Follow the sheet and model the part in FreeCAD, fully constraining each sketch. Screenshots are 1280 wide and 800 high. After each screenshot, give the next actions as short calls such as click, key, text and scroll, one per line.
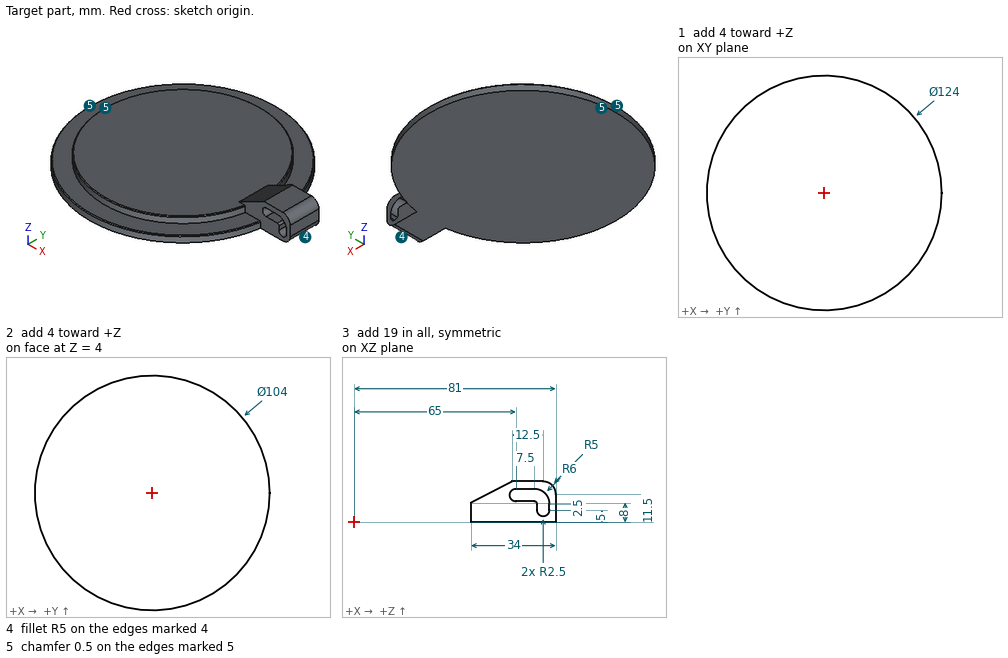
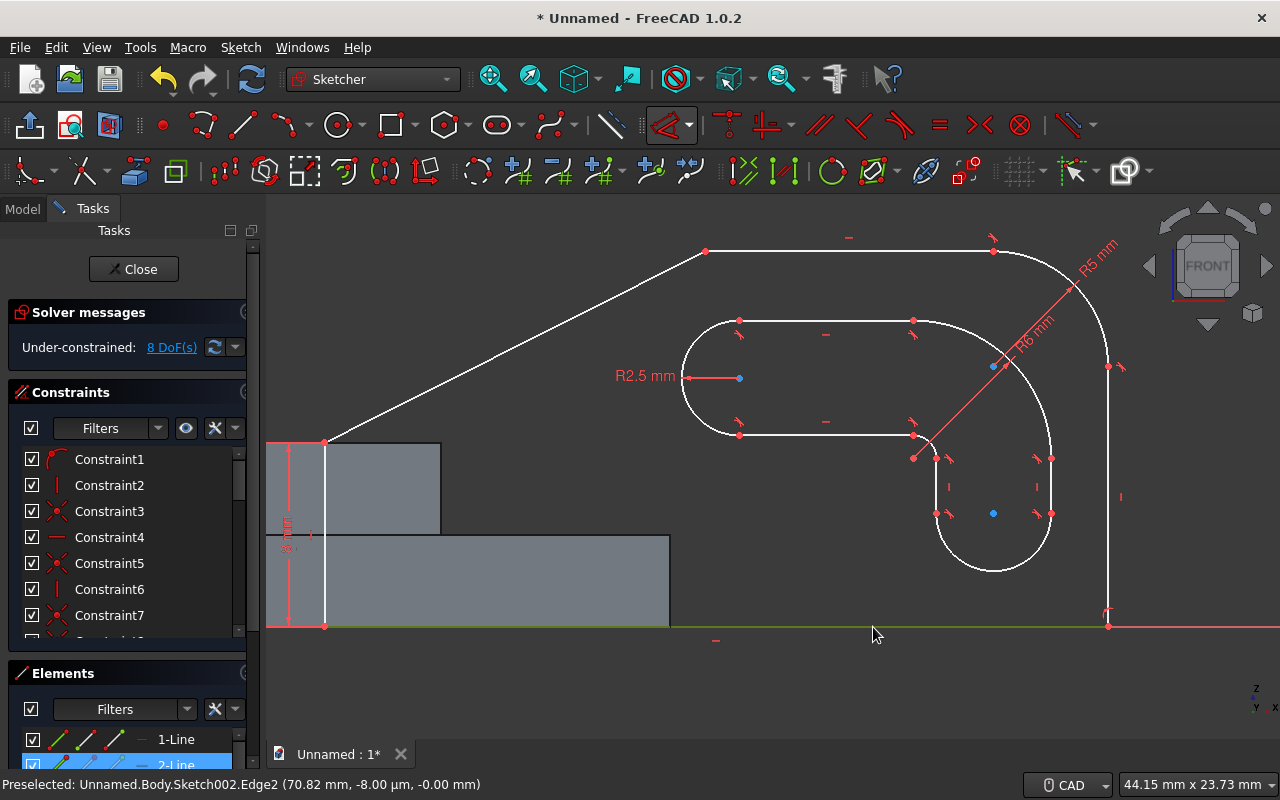
key(l)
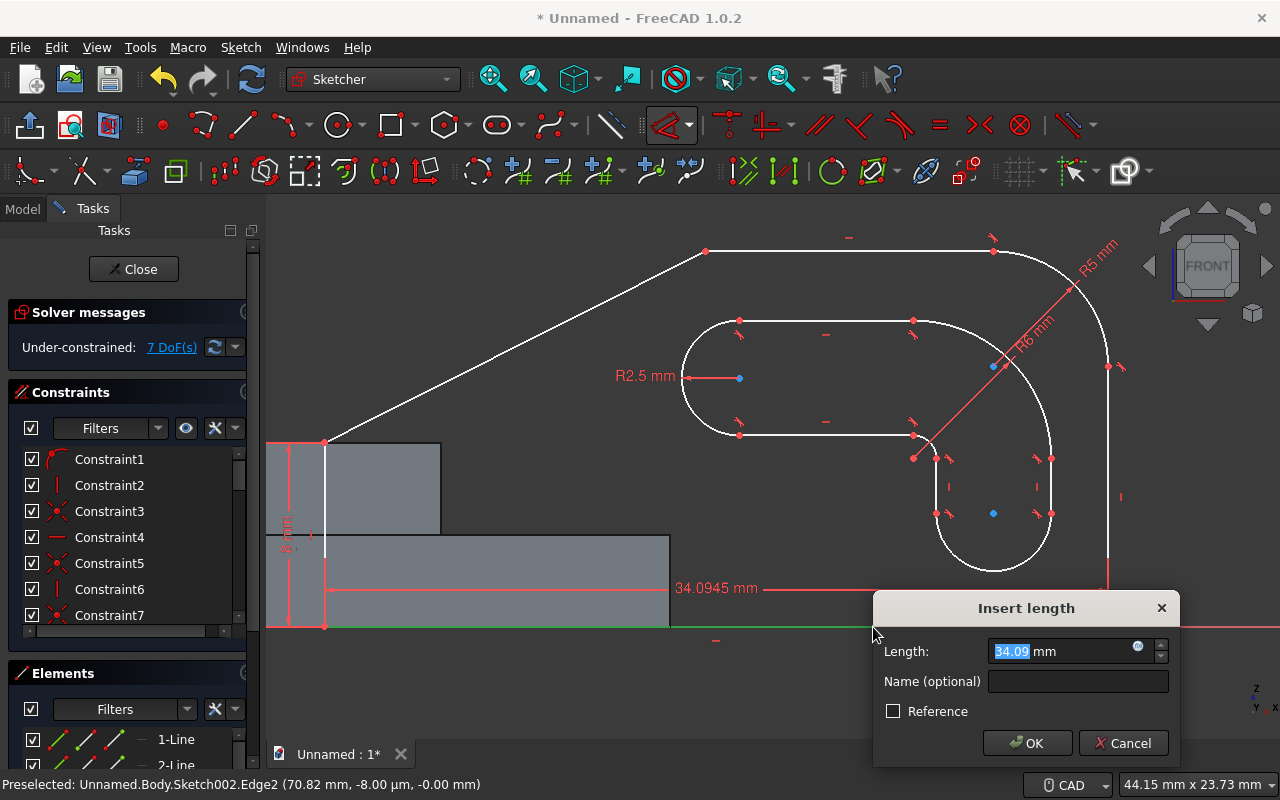
text(34)
key(Return)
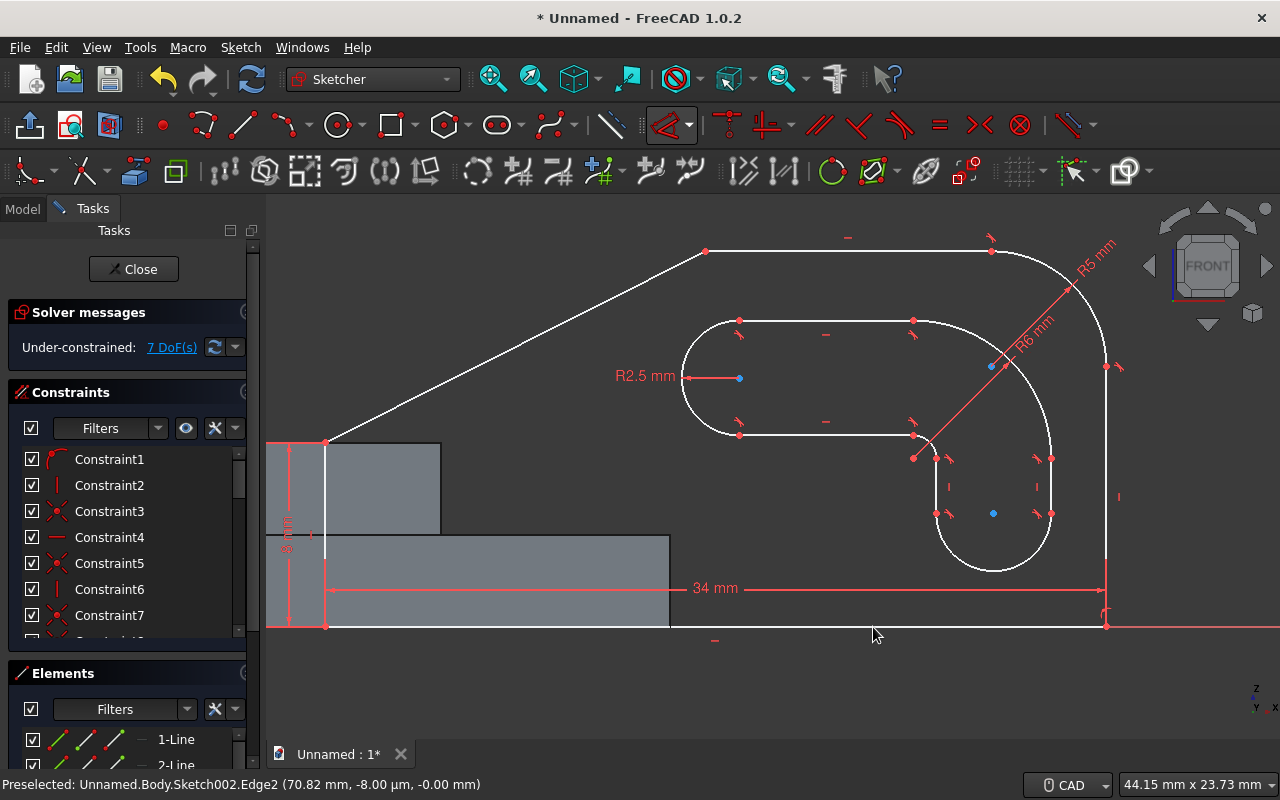
click(1051, 514)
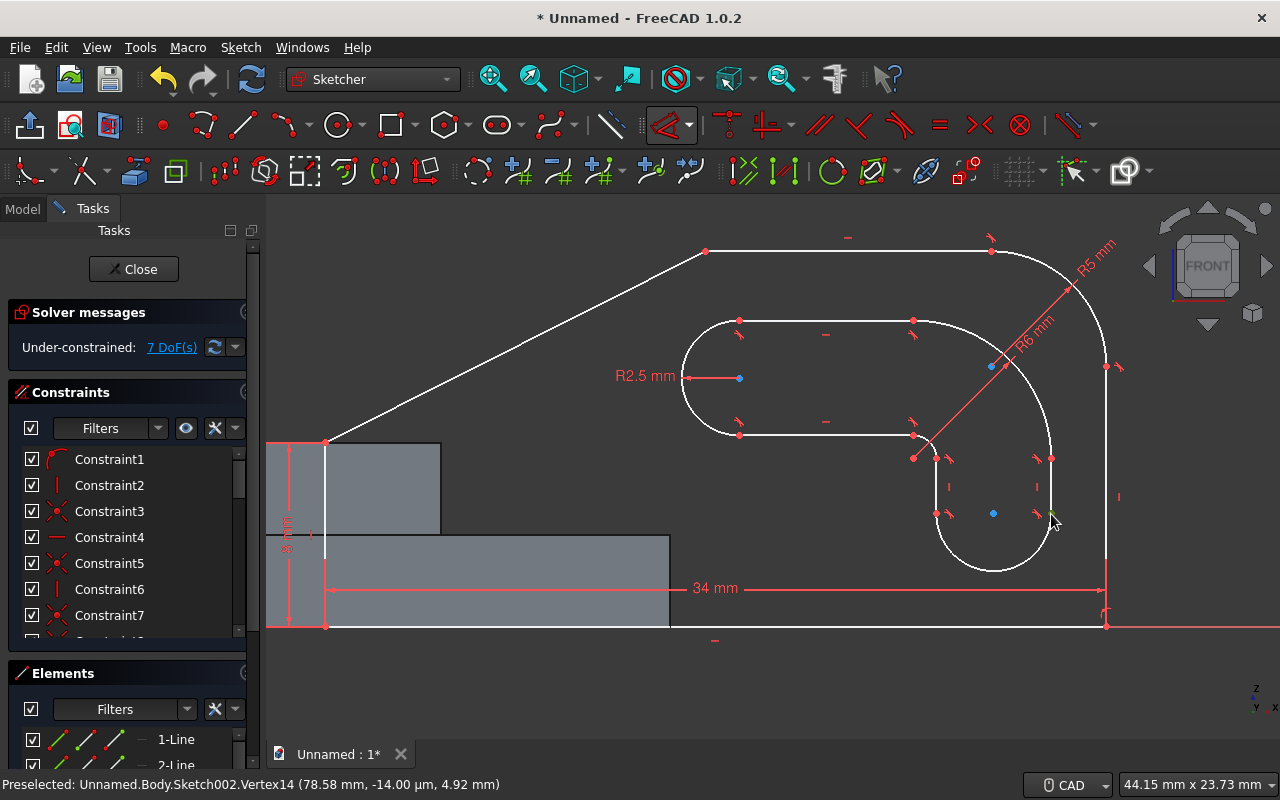
click(692, 126)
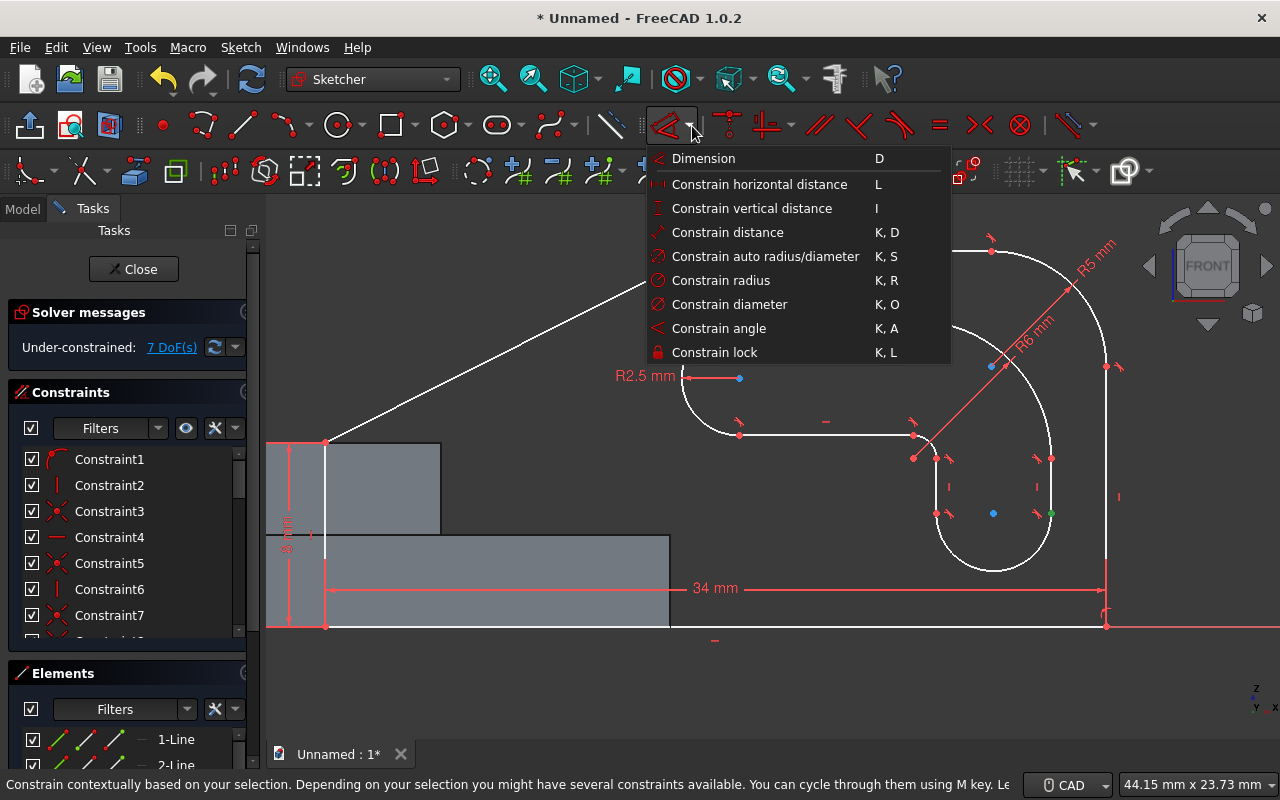
click(799, 208)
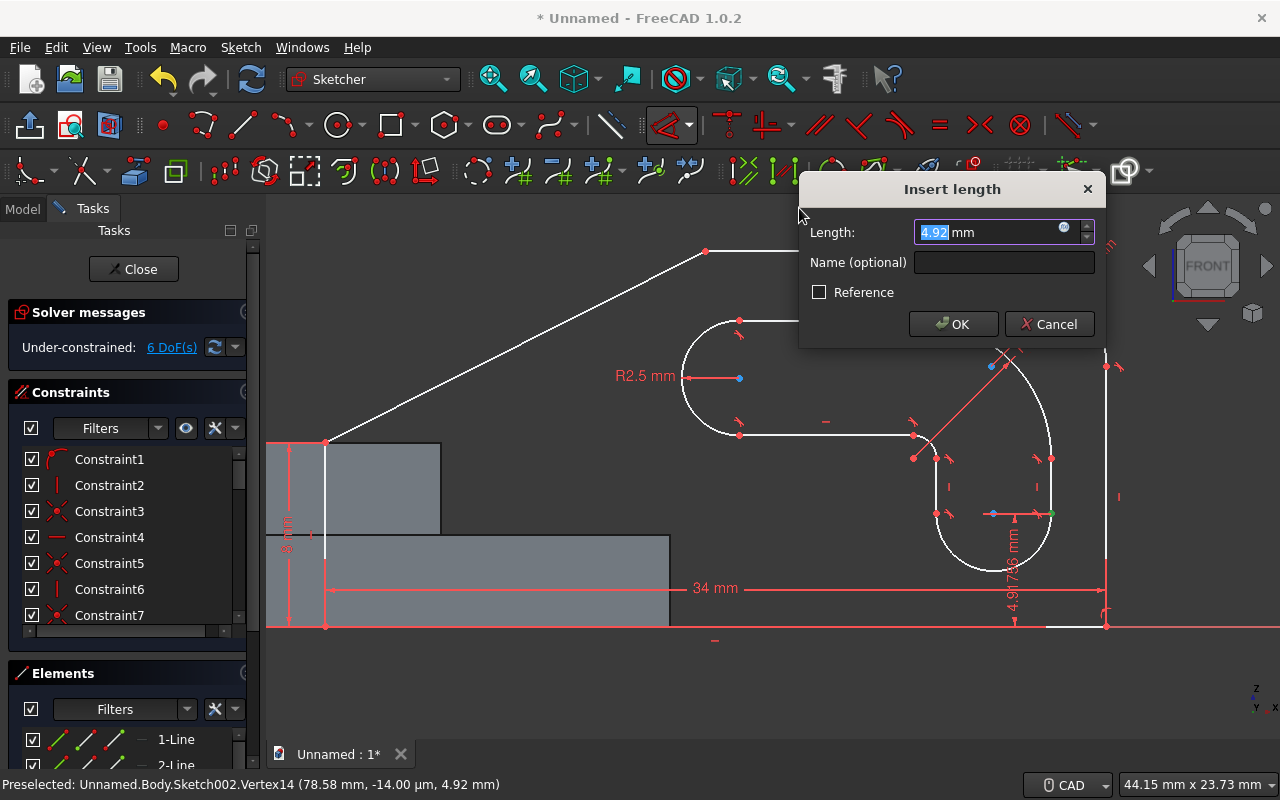
text(5)
key(Return)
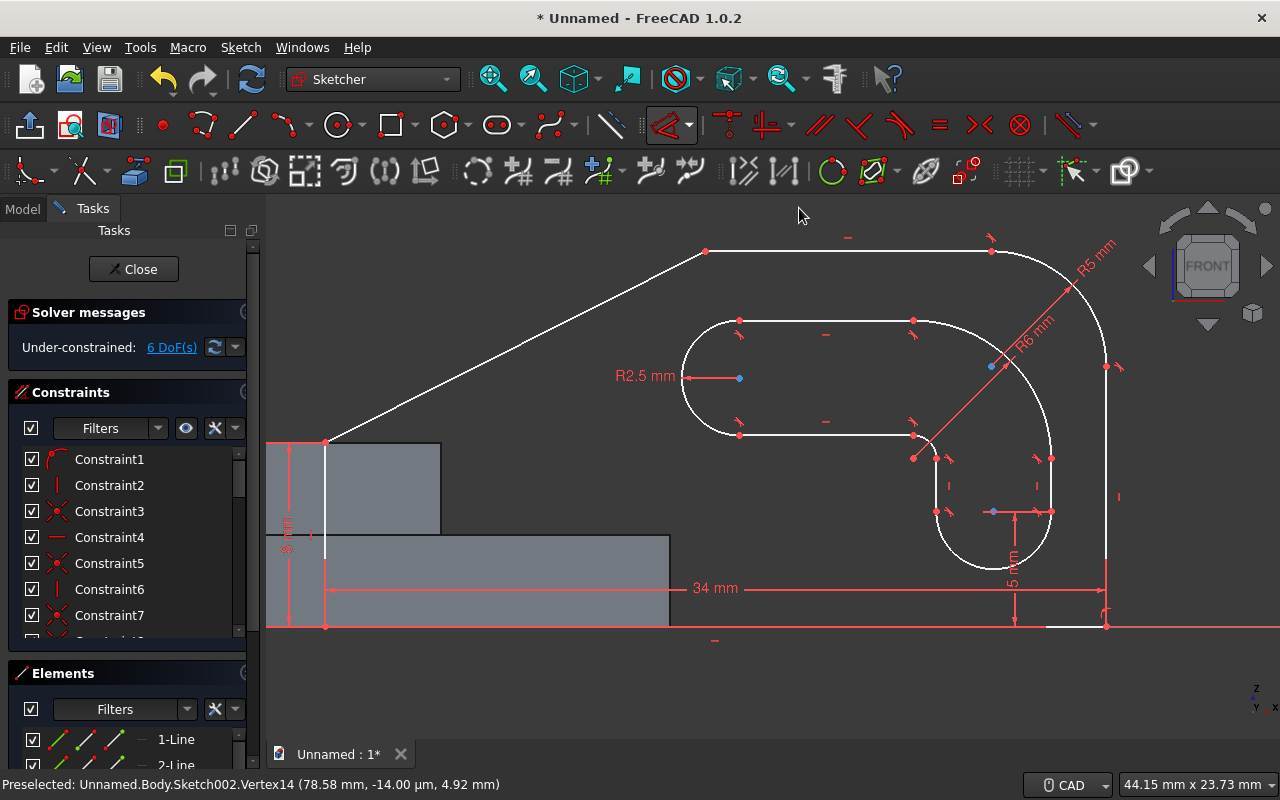
click(1051, 496)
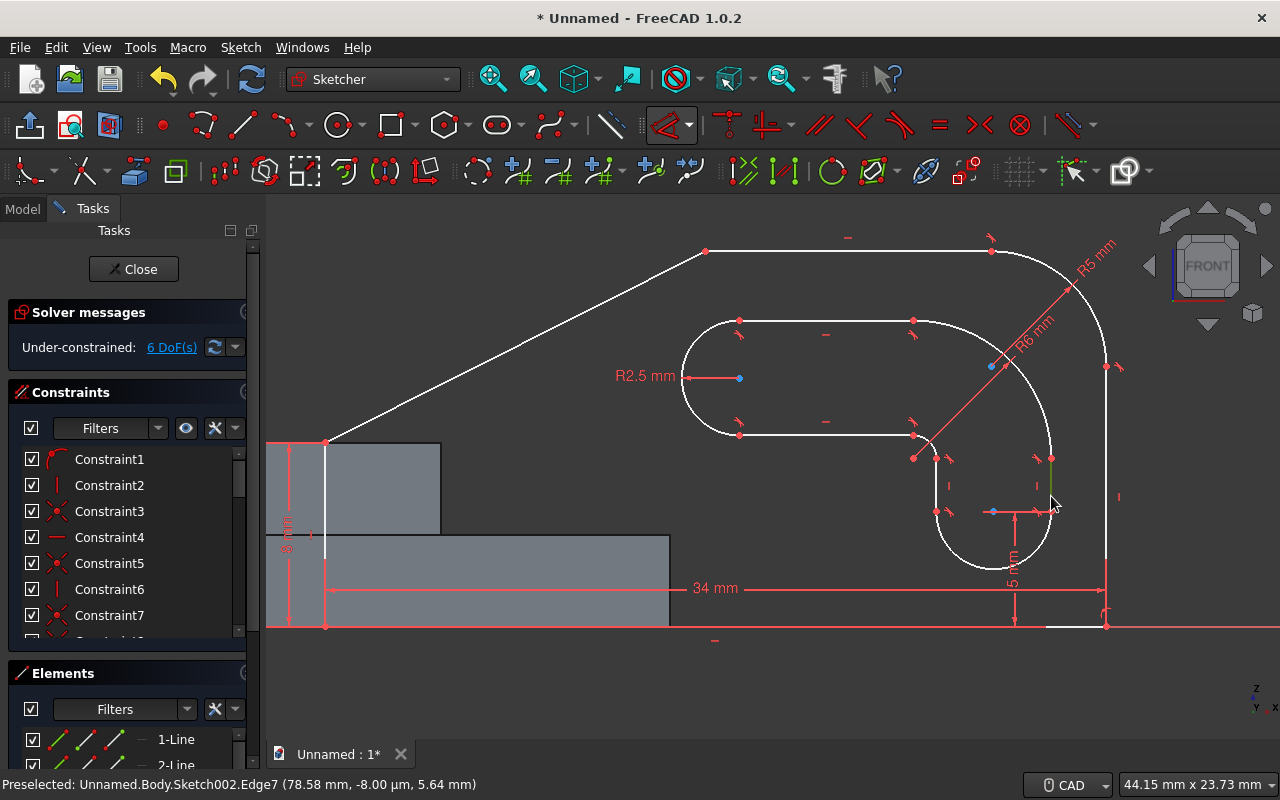
click(692, 126)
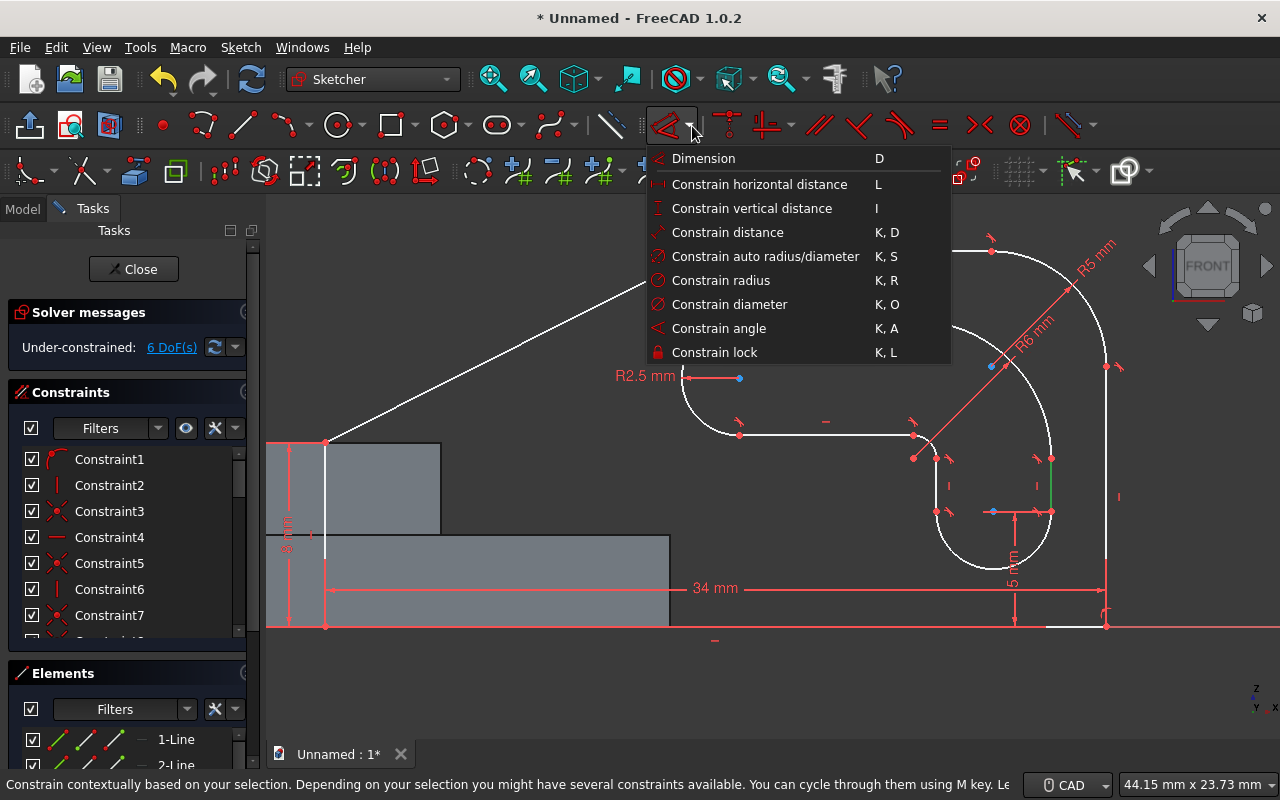
click(799, 208)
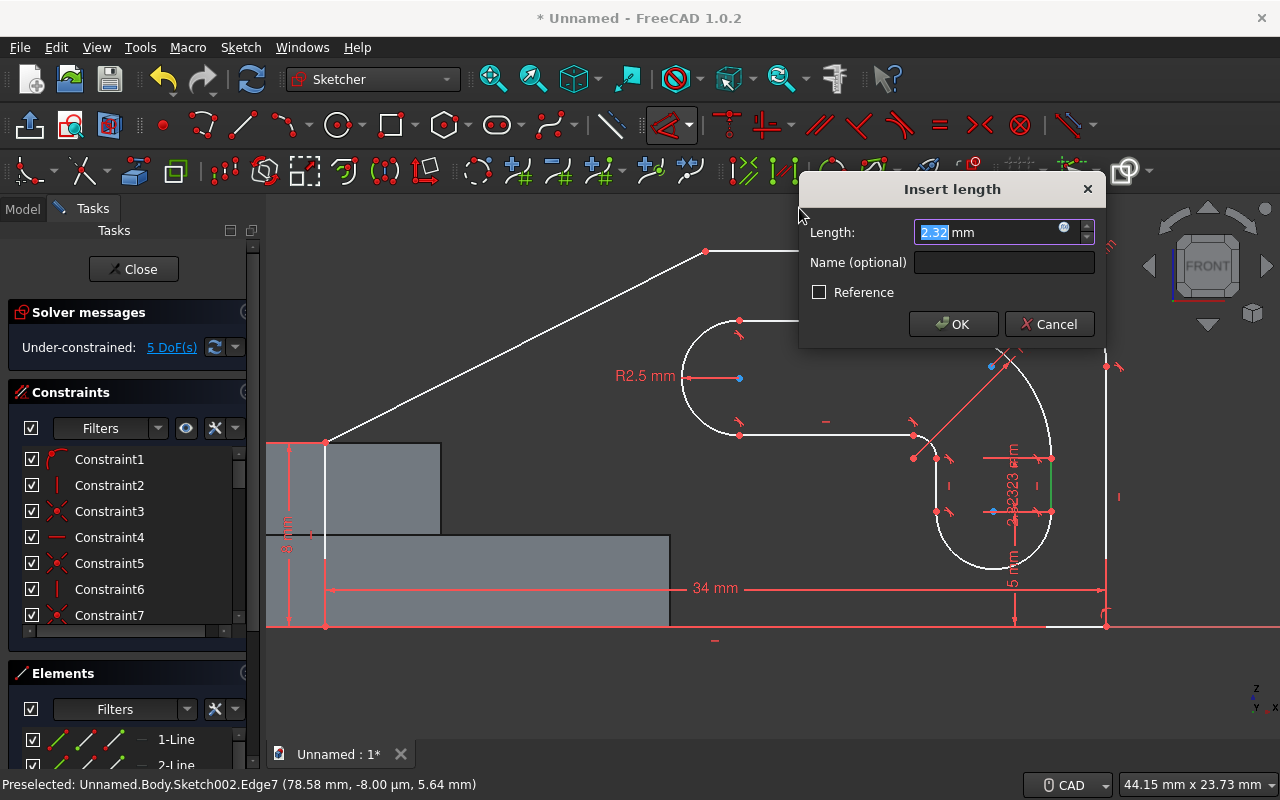
text(2.5)
key(Return)